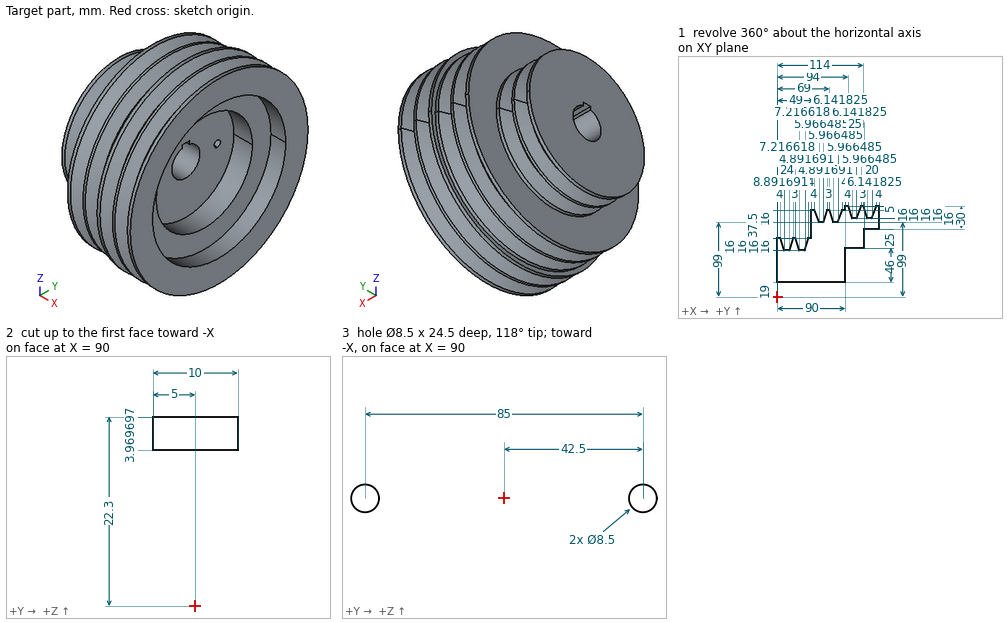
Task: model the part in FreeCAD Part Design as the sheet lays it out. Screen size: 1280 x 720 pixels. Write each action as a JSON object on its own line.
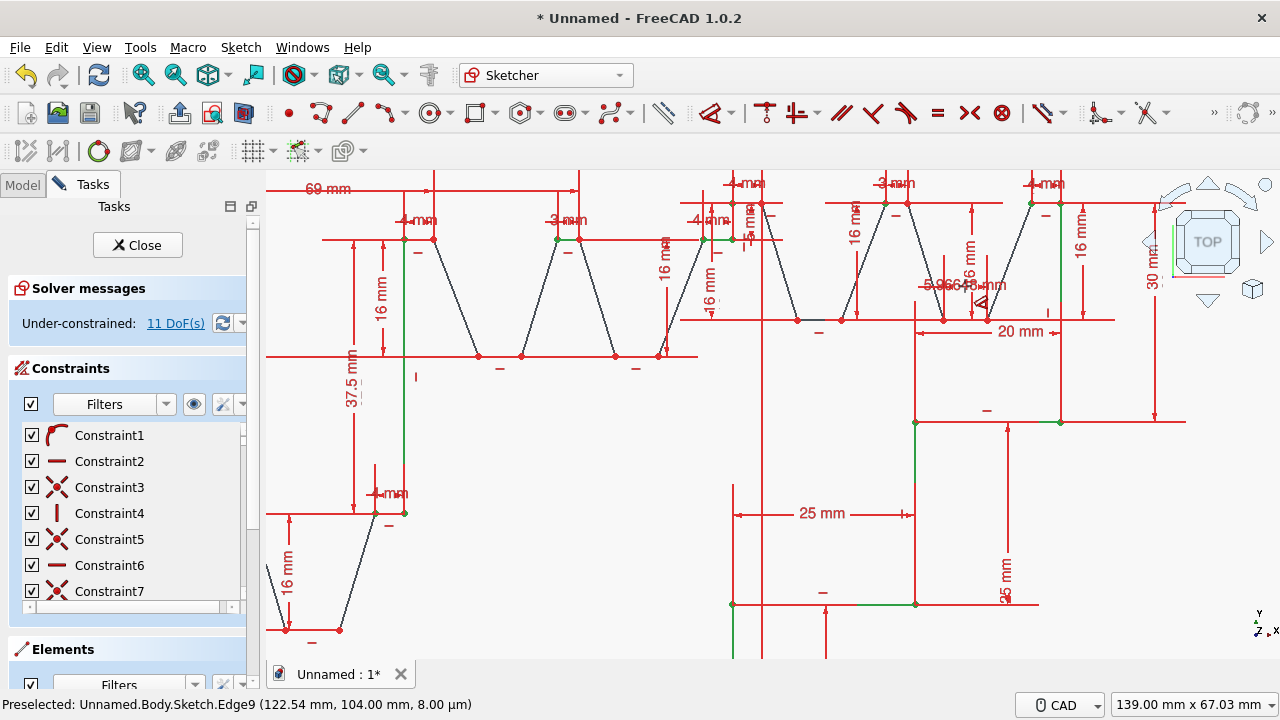
{"action": "left_click", "coordinate": [828, 320]}
{"action": "left_click", "coordinate": [820, 286]}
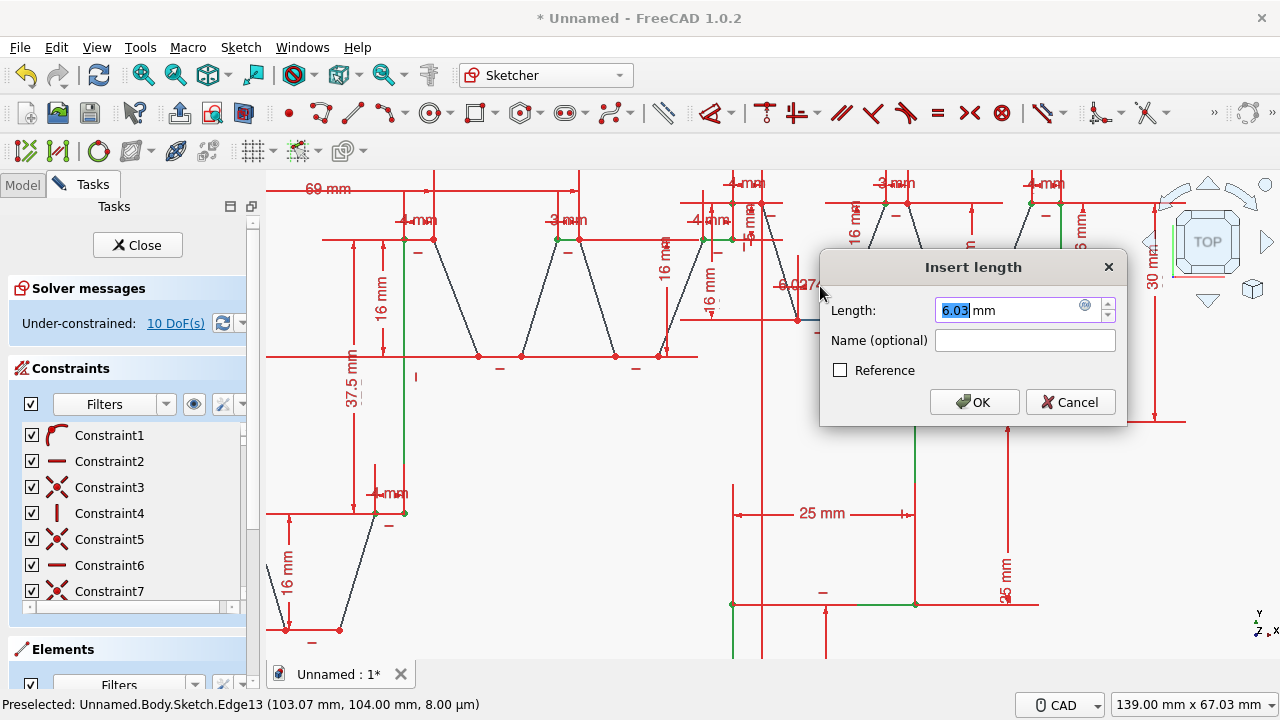
{"action": "type", "text": "5.966485"}
{"action": "key", "text": "Return"}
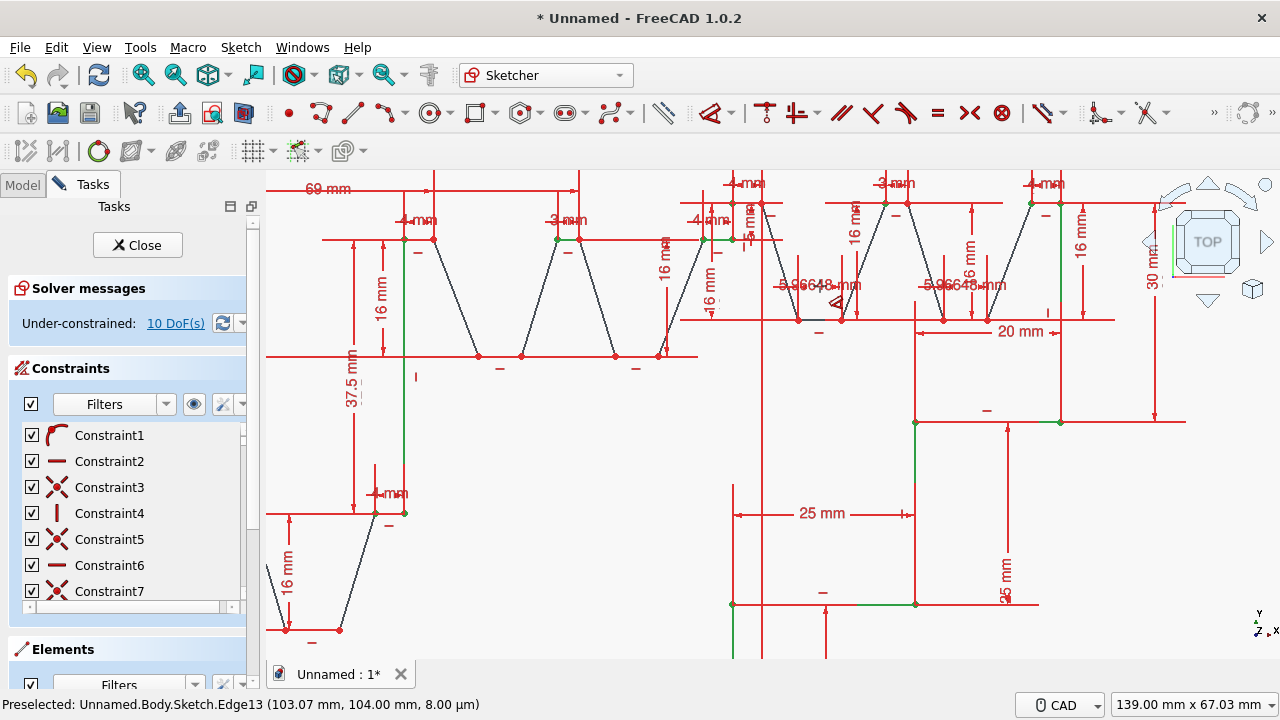
{"action": "left_click", "coordinate": [645, 357]}
{"action": "left_click", "coordinate": [637, 323]}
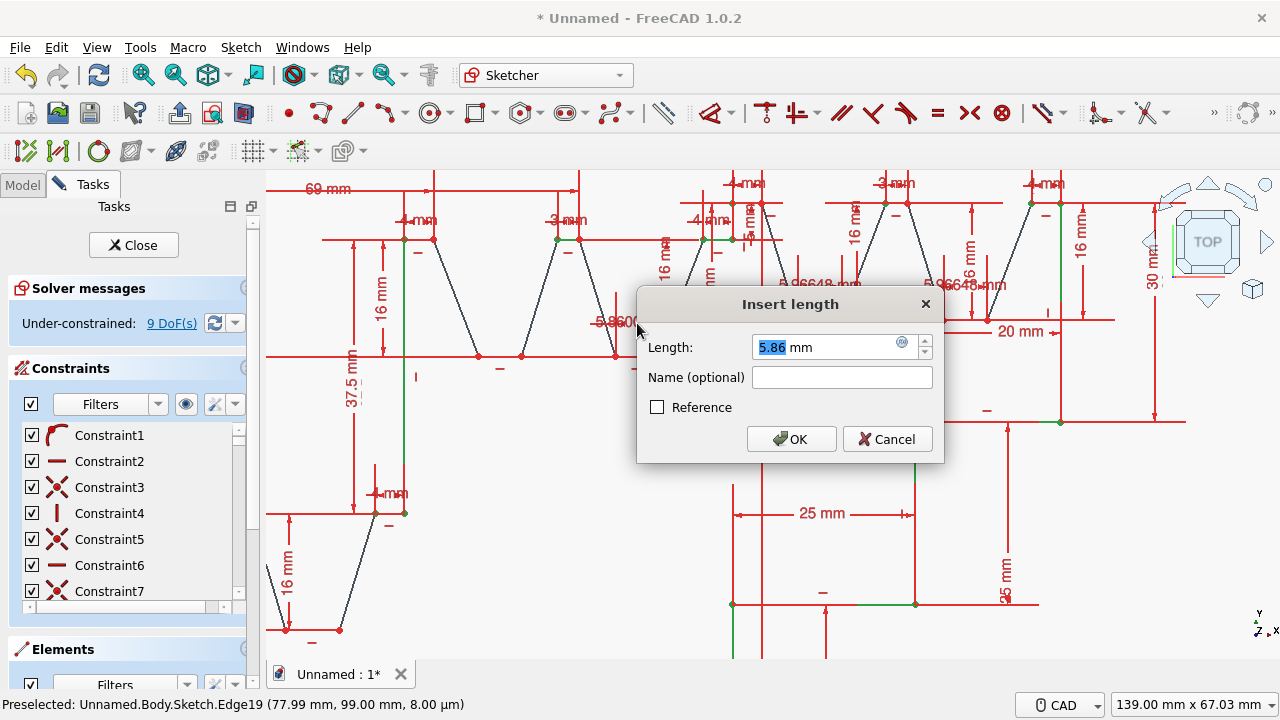
{"action": "type", "text": "5.966485"}
{"action": "key", "text": "Return"}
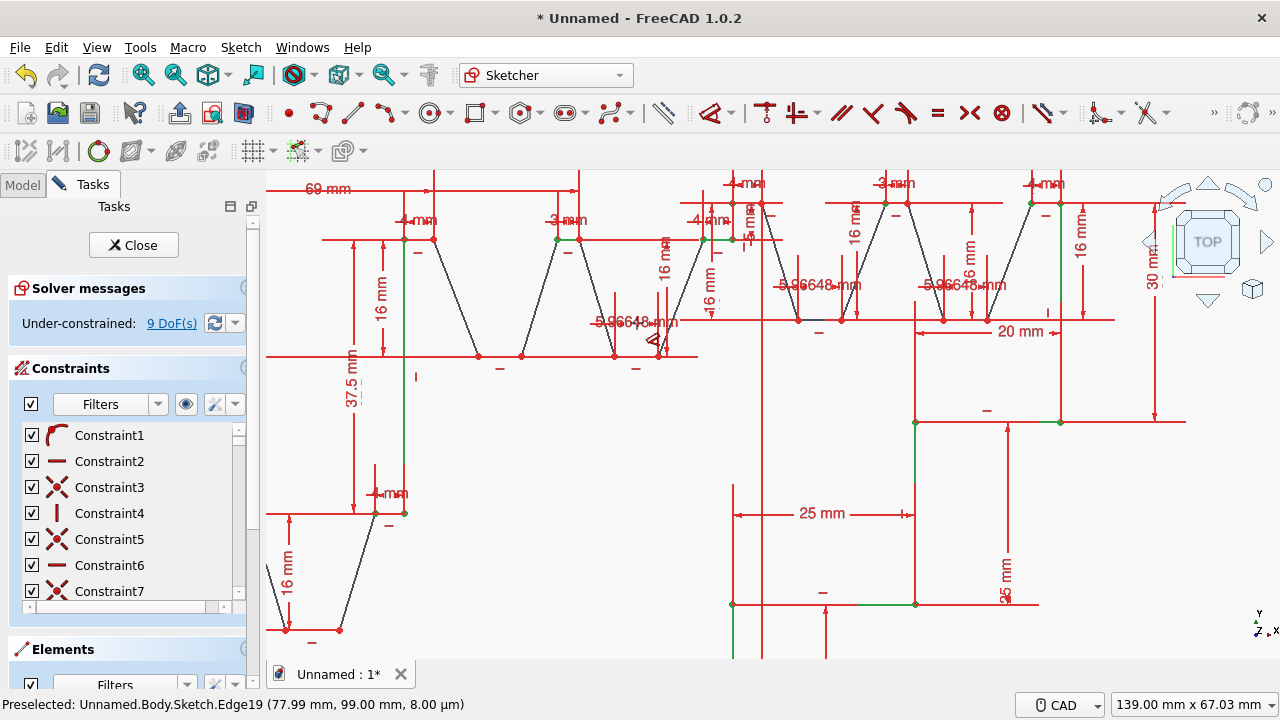
{"action": "left_click", "coordinate": [509, 357]}
{"action": "left_click", "coordinate": [500, 323]}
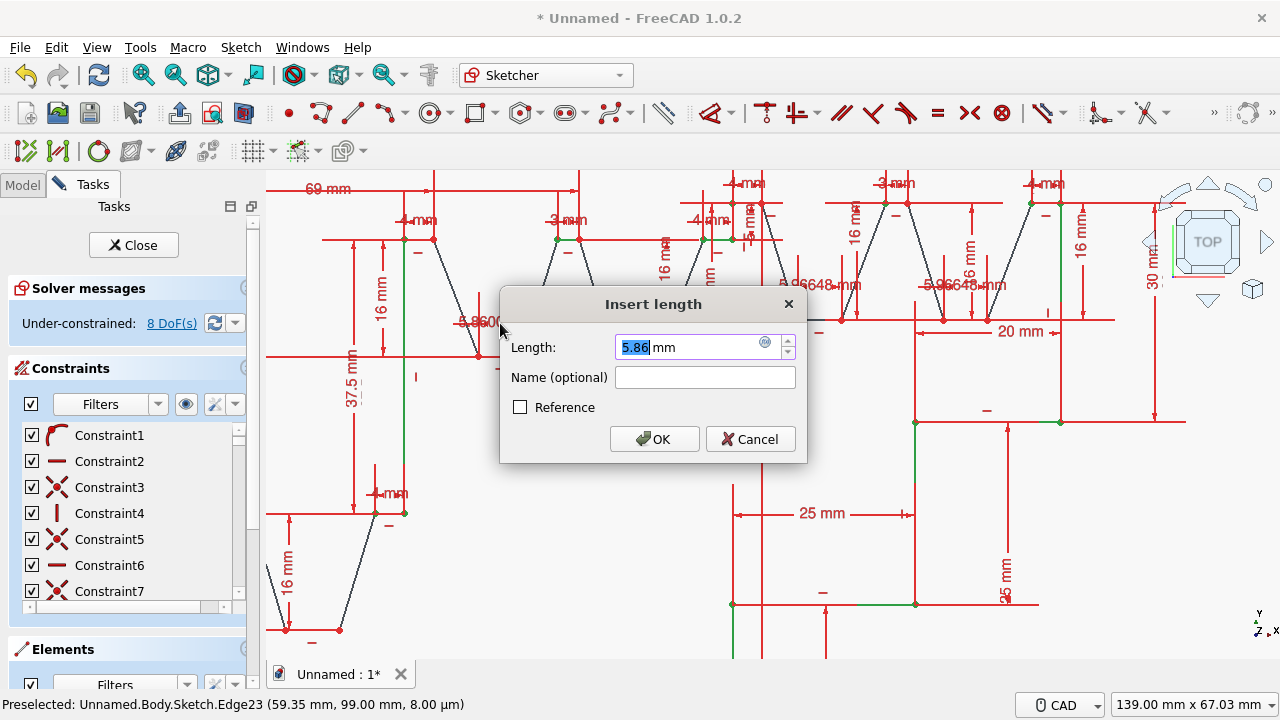
{"action": "type", "text": "5.966485"}
{"action": "key", "text": "Return"}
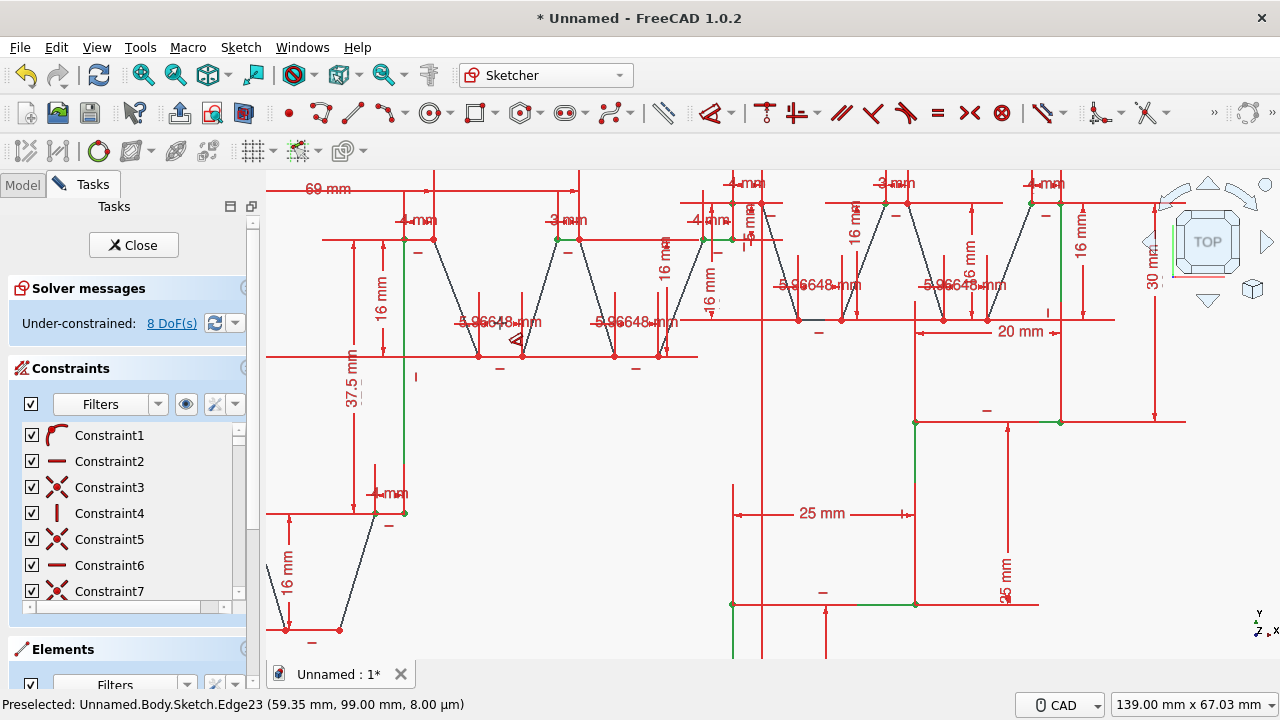
{"action": "left_click", "coordinate": [323, 630]}
{"action": "left_click", "coordinate": [317, 596]}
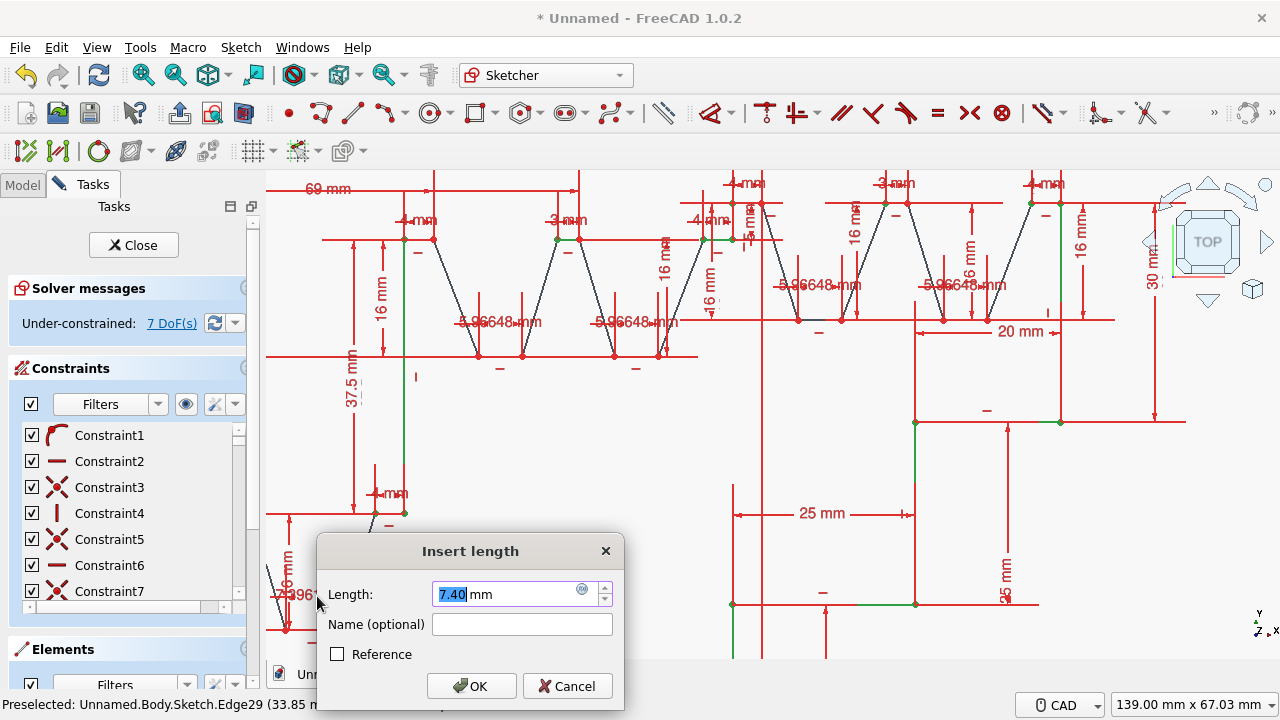
{"action": "type", "text": "7.216618"}
{"action": "key", "text": "Return"}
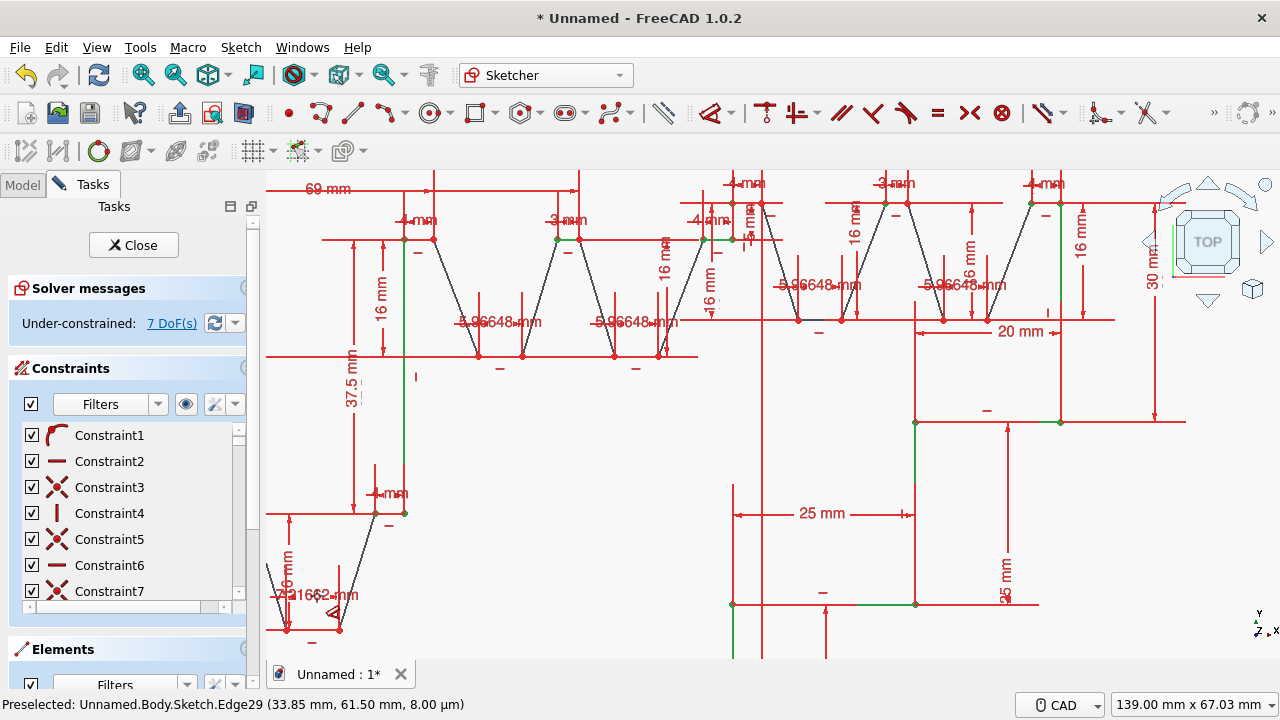
{"action": "scroll", "coordinate": [784, 283], "scroll_direction": "down", "scroll_amount": 5}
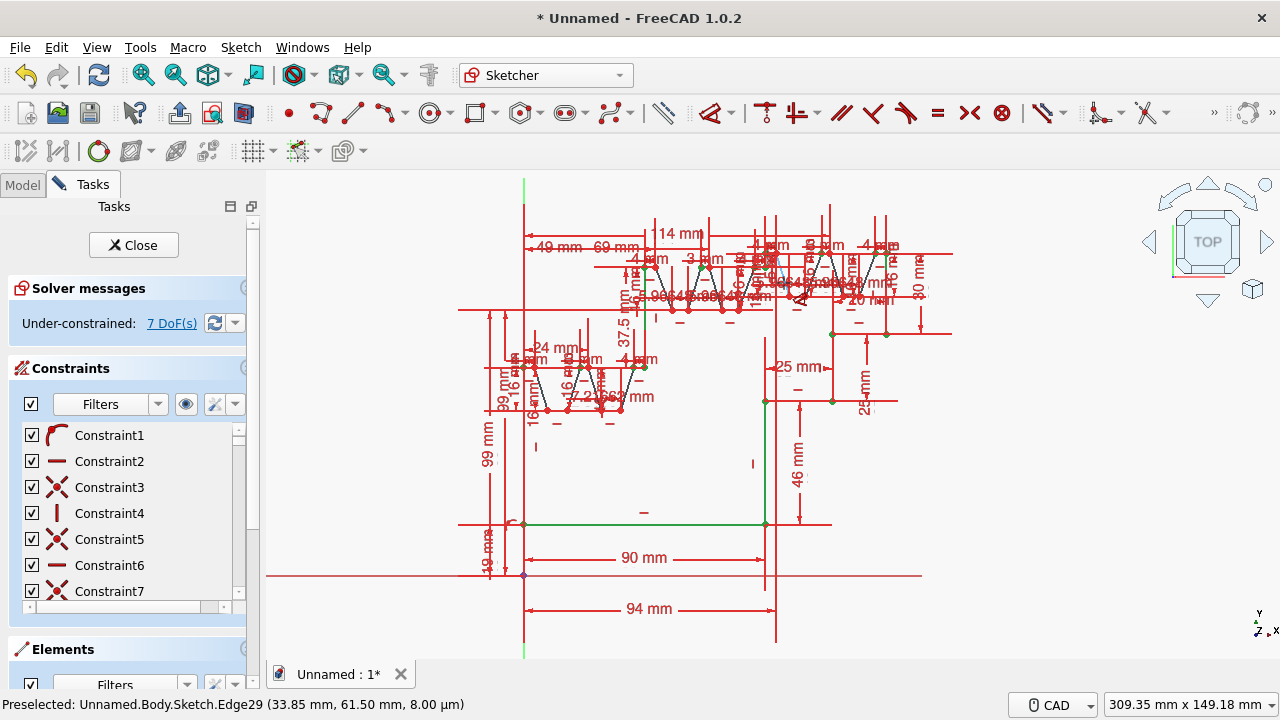
{"action": "scroll", "coordinate": [561, 411], "scroll_direction": "up", "scroll_amount": 5}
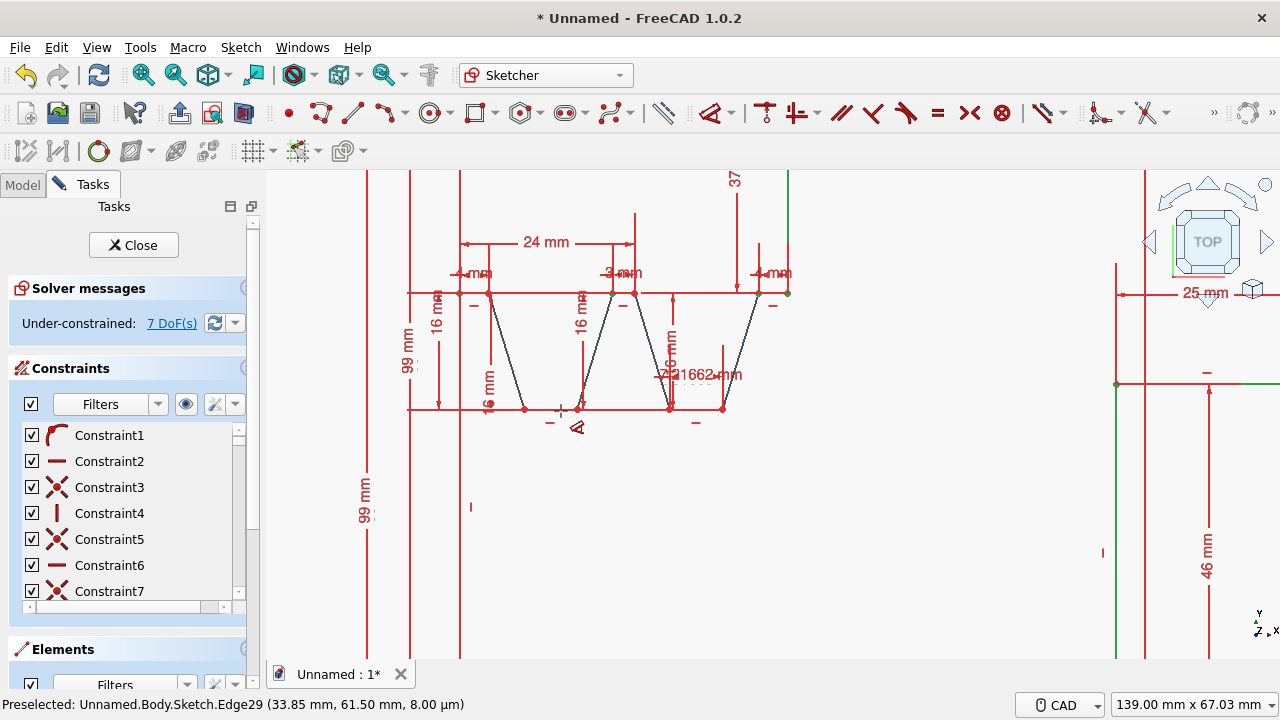
{"action": "left_click", "coordinate": [561, 410]}
{"action": "left_click", "coordinate": [563, 376]}